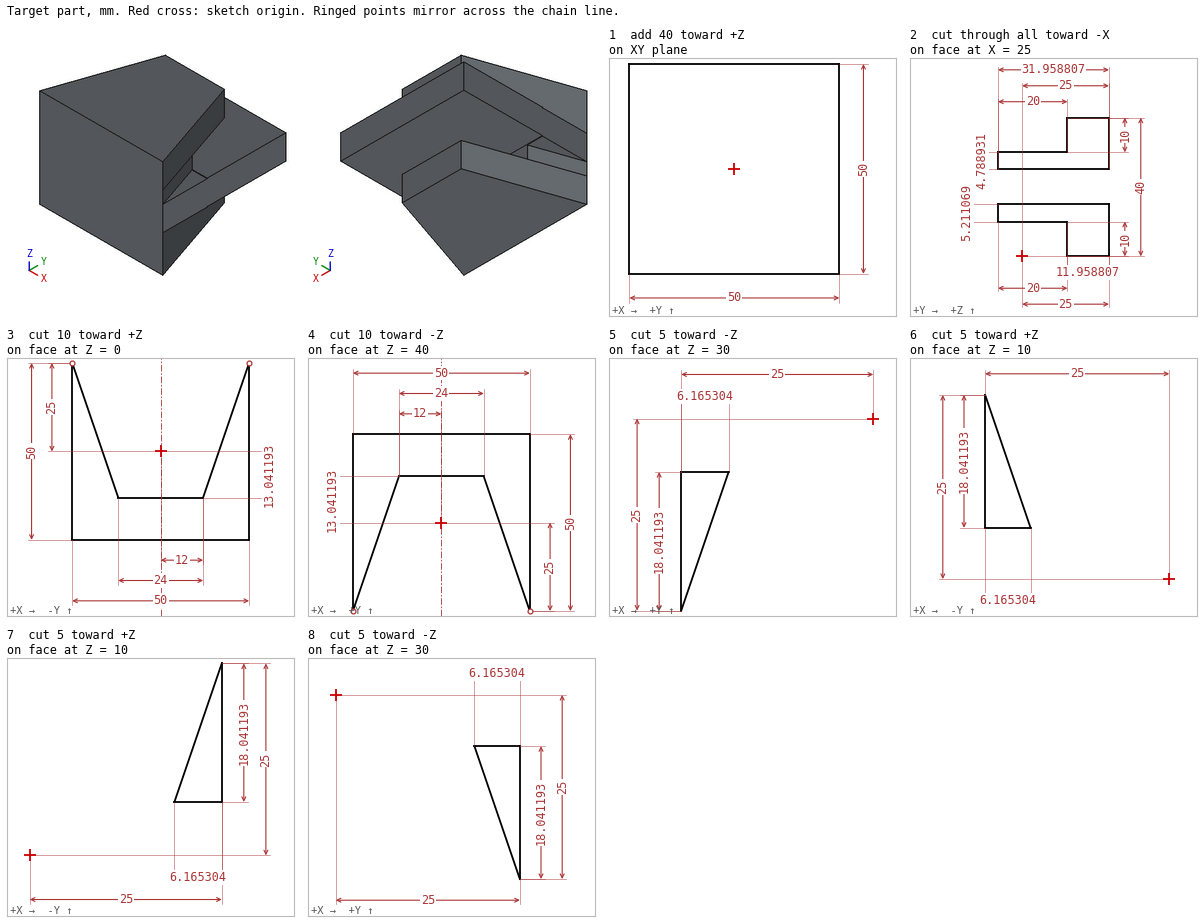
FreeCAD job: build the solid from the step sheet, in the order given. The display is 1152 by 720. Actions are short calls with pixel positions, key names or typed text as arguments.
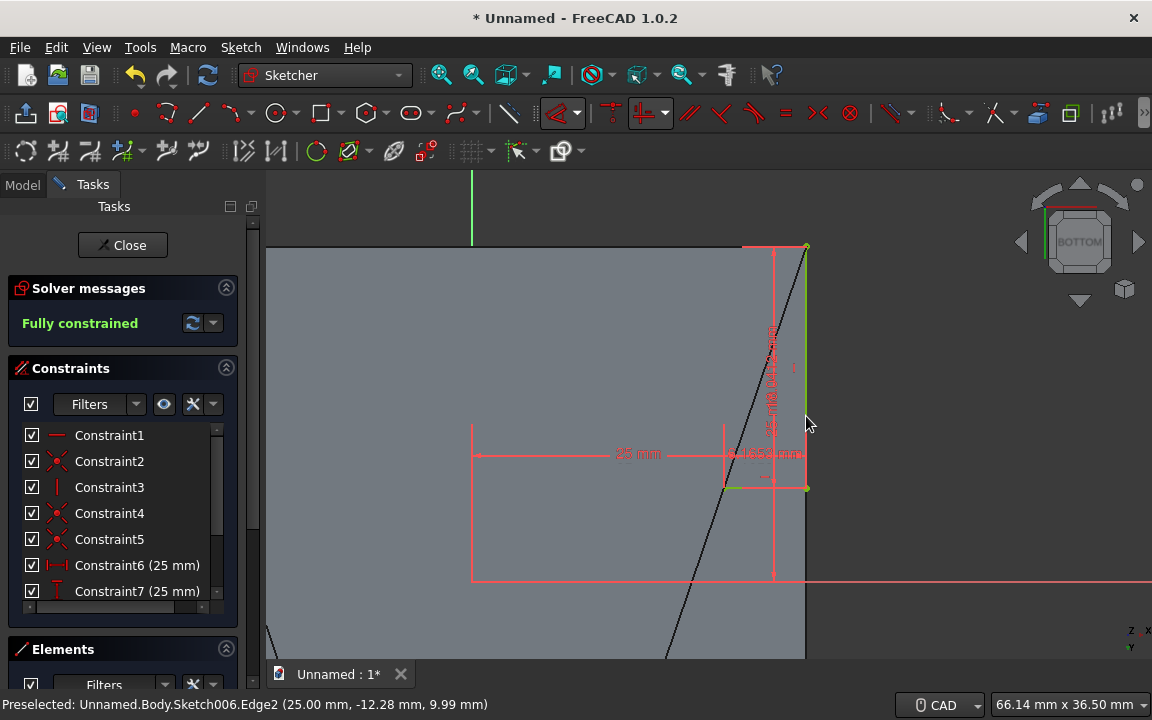
click(123, 245)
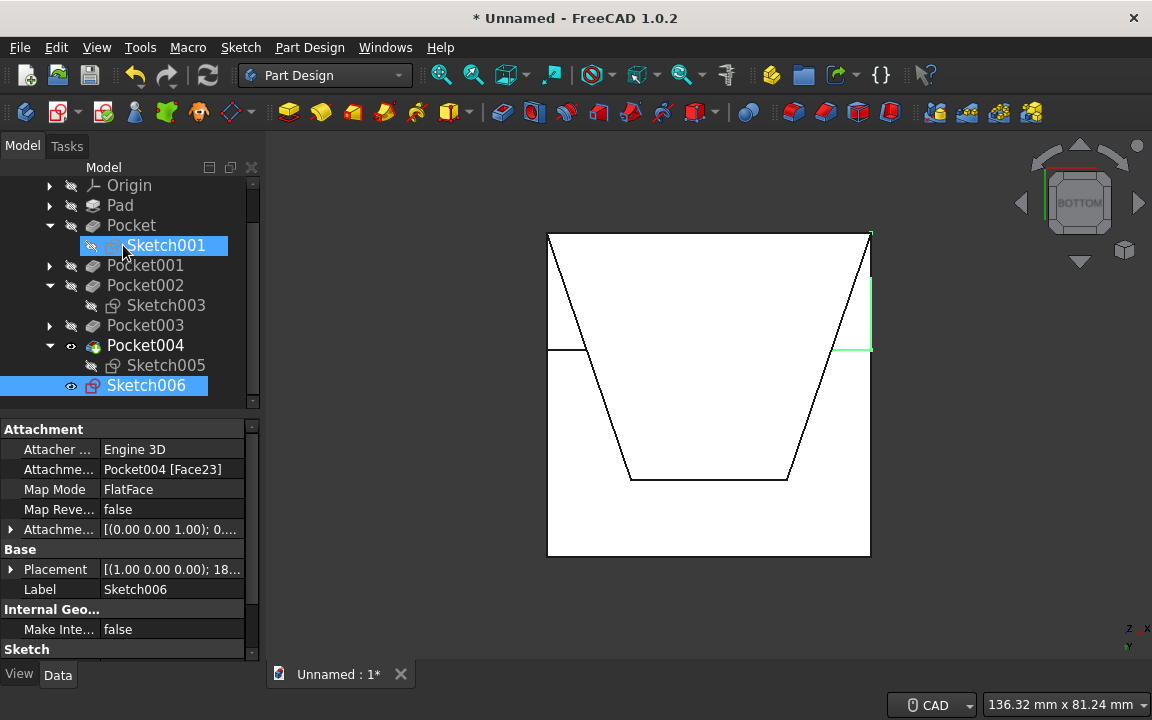
click(504, 112)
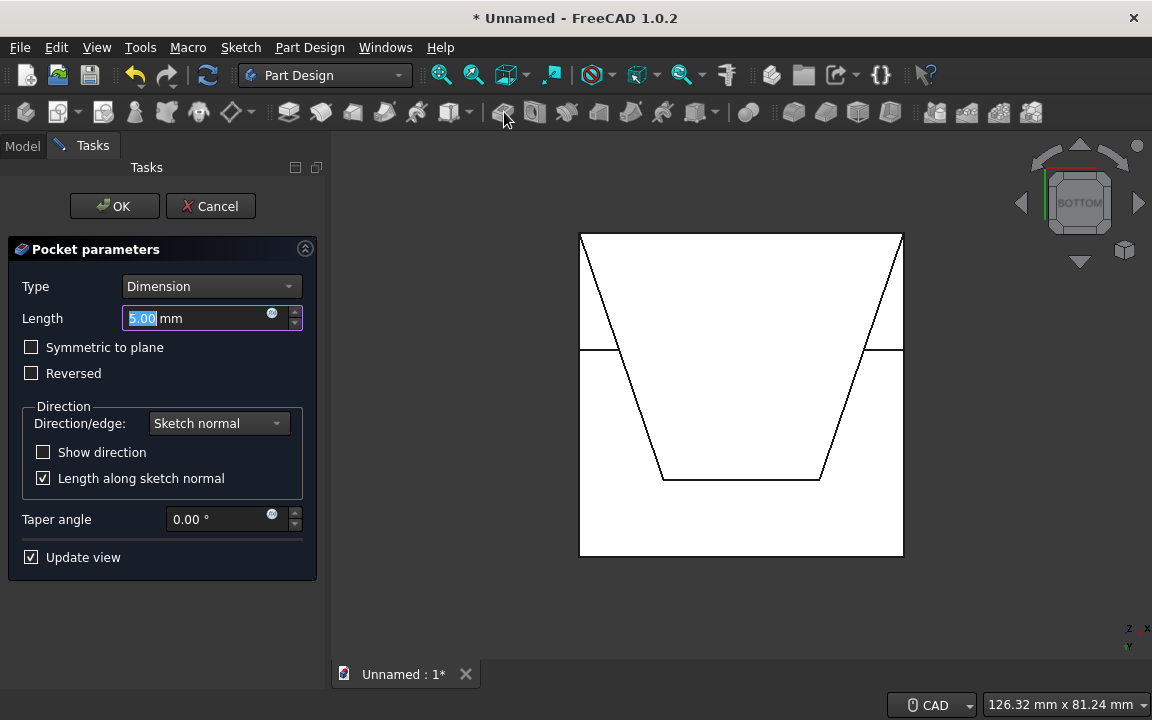
text(5)
key(Tab)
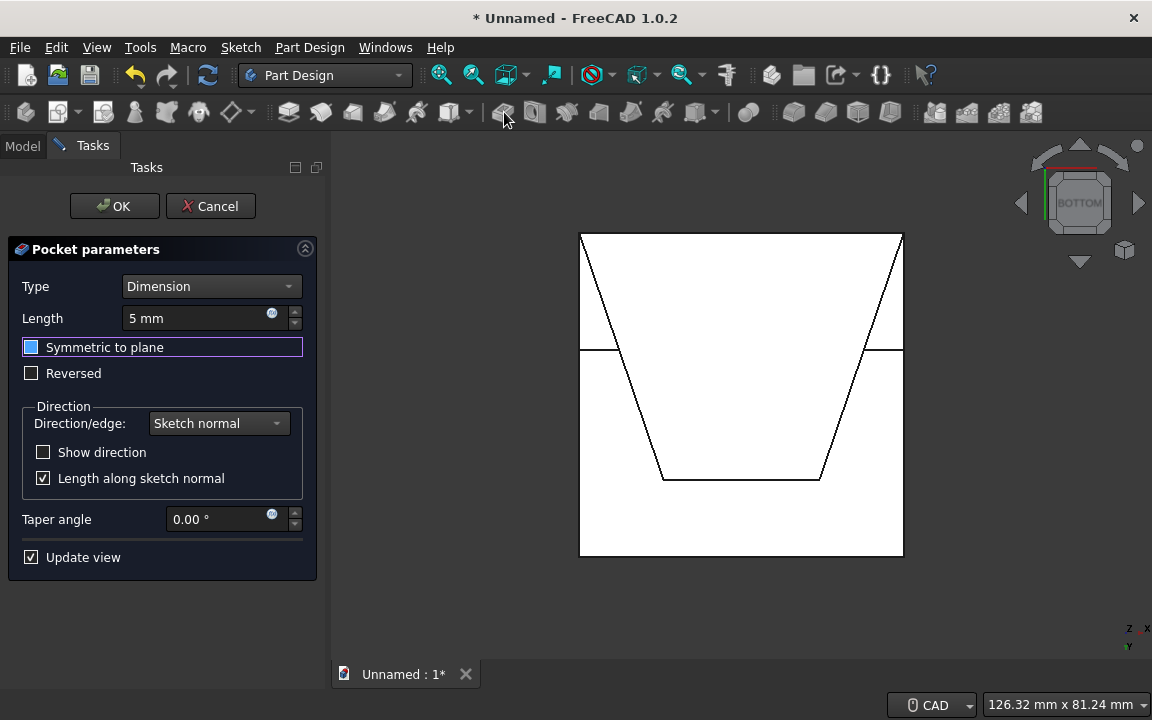
click(115, 206)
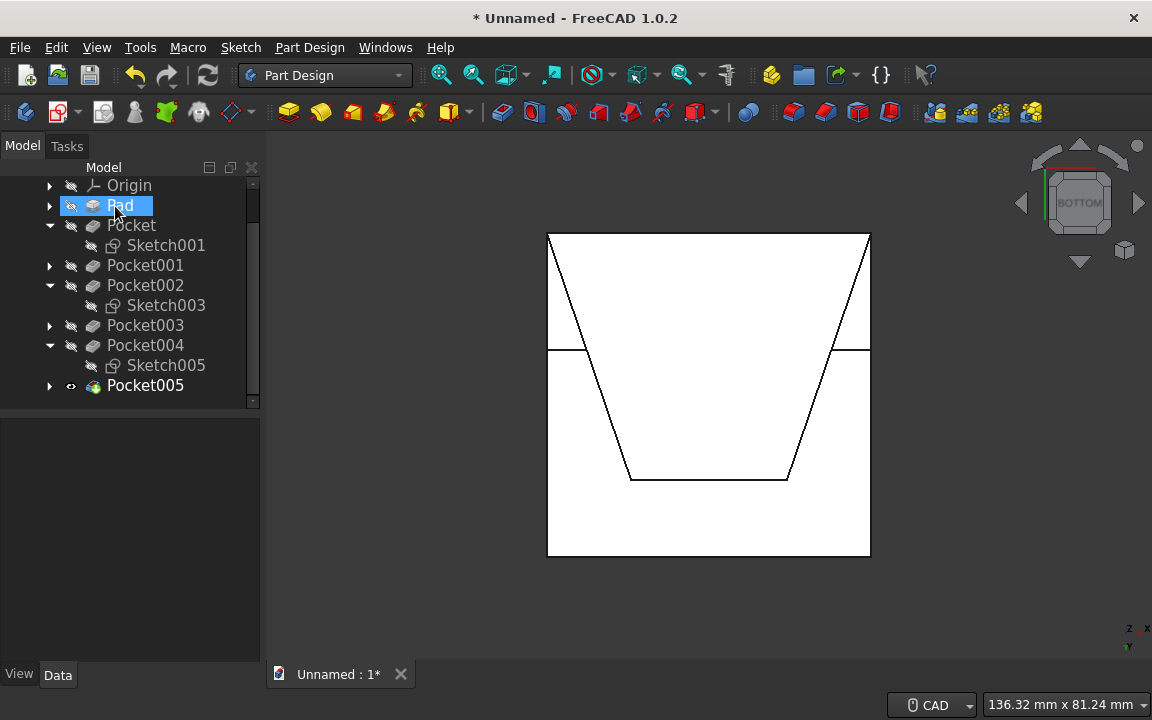
key(0)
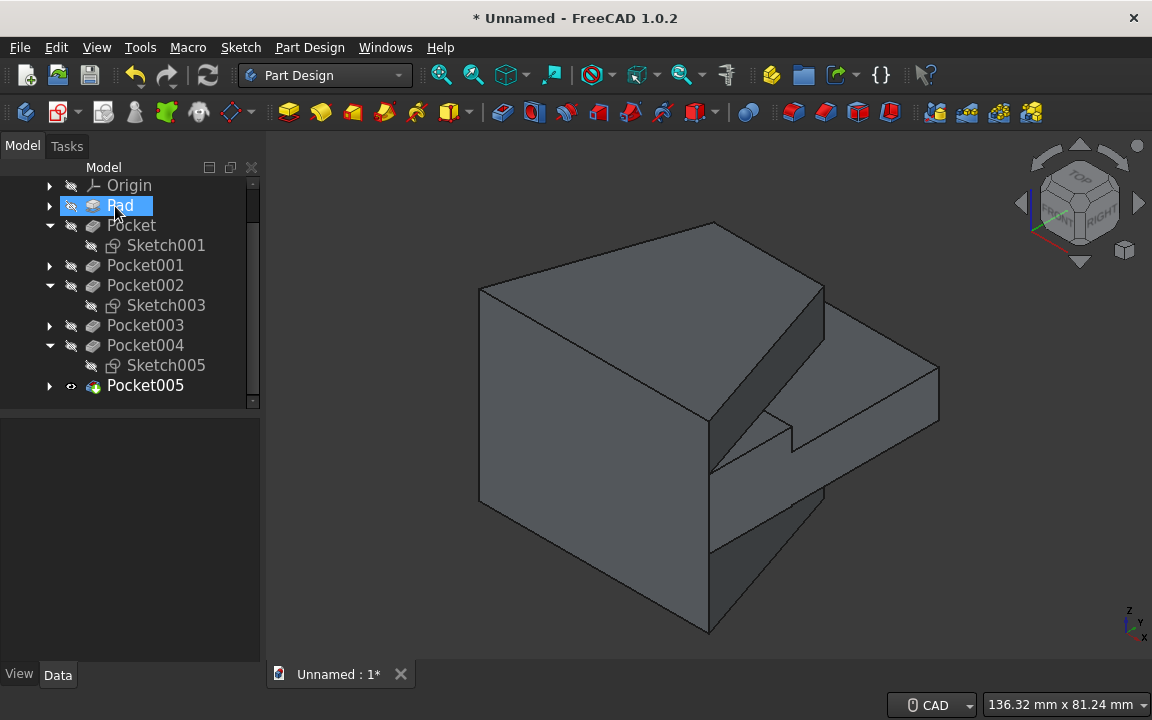
click(764, 430)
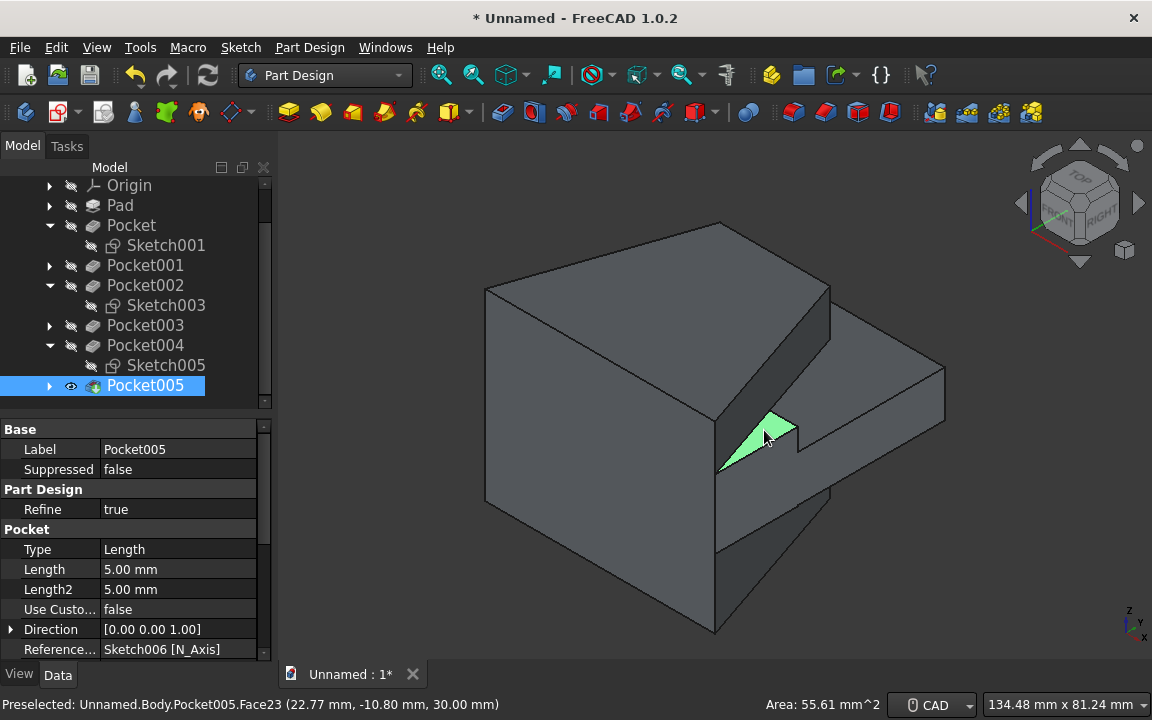
click(58, 112)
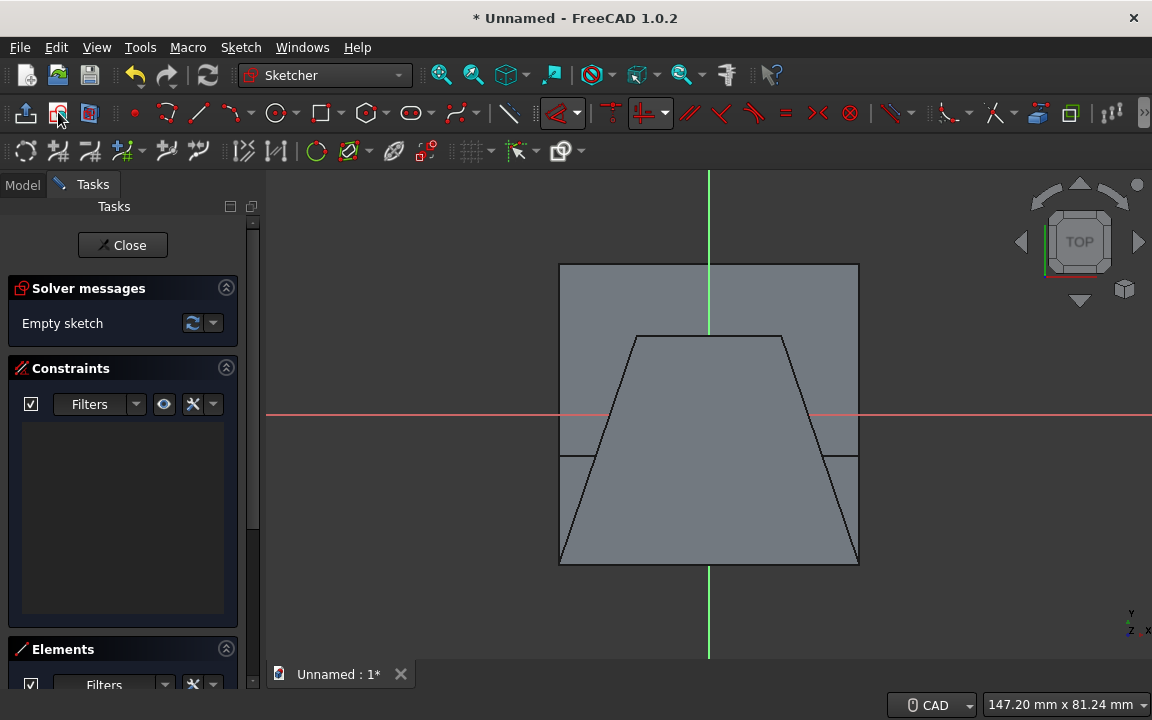
key(q)
key(s)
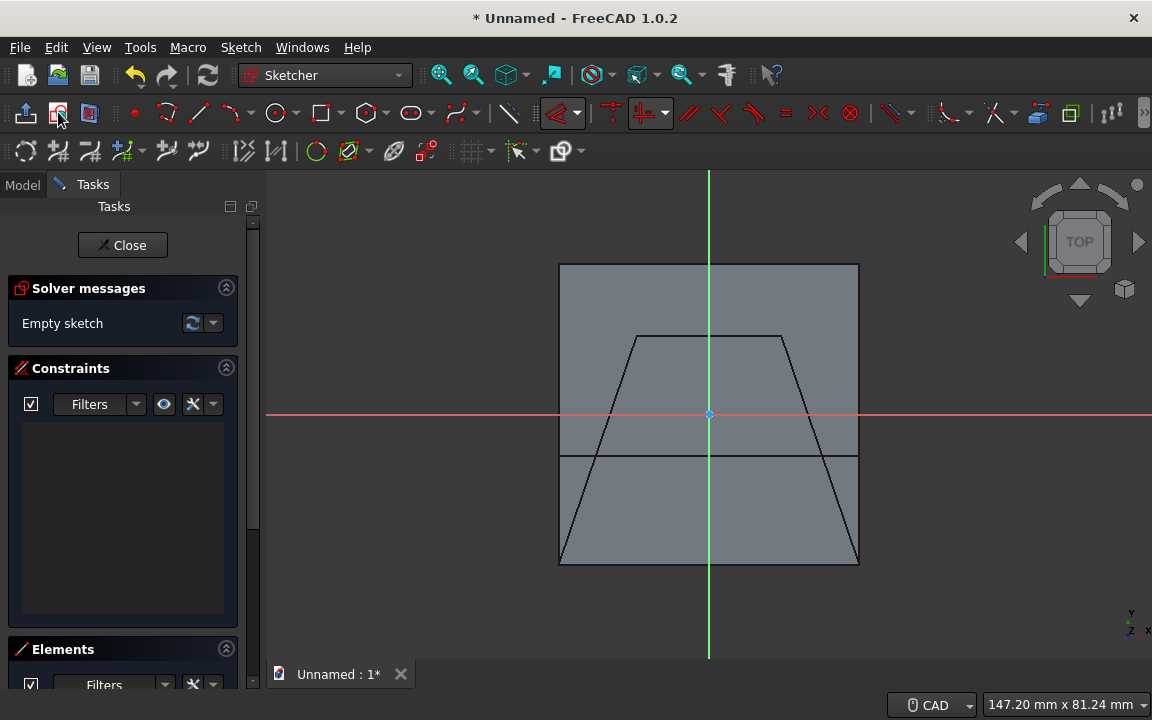
scroll(902, 551, up, 4)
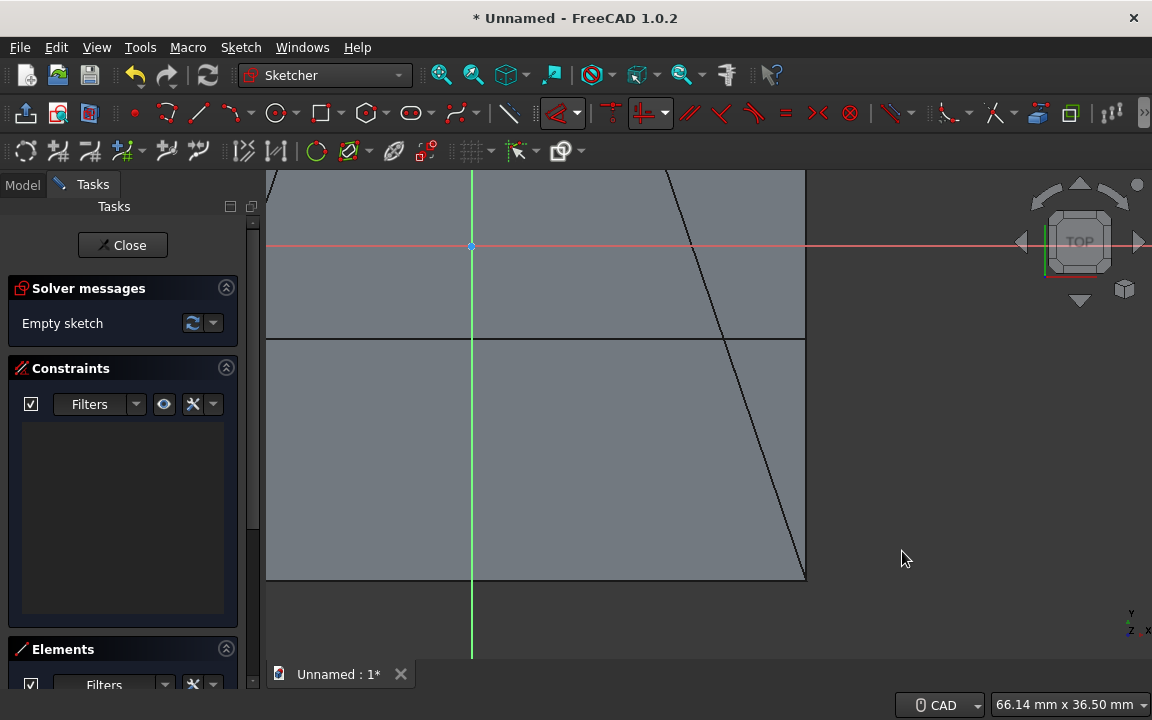
key(g)
key(m)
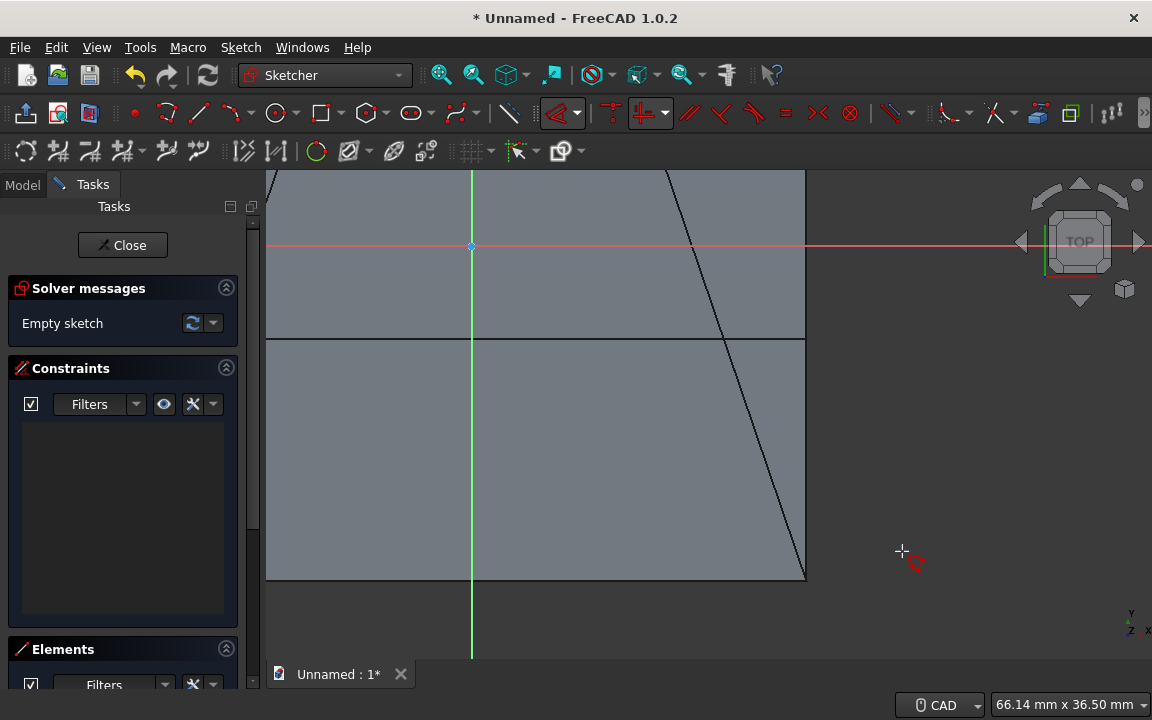
click(724, 339)
click(806, 581)
click(806, 339)
click(724, 340)
key(Escape)
key(Escape)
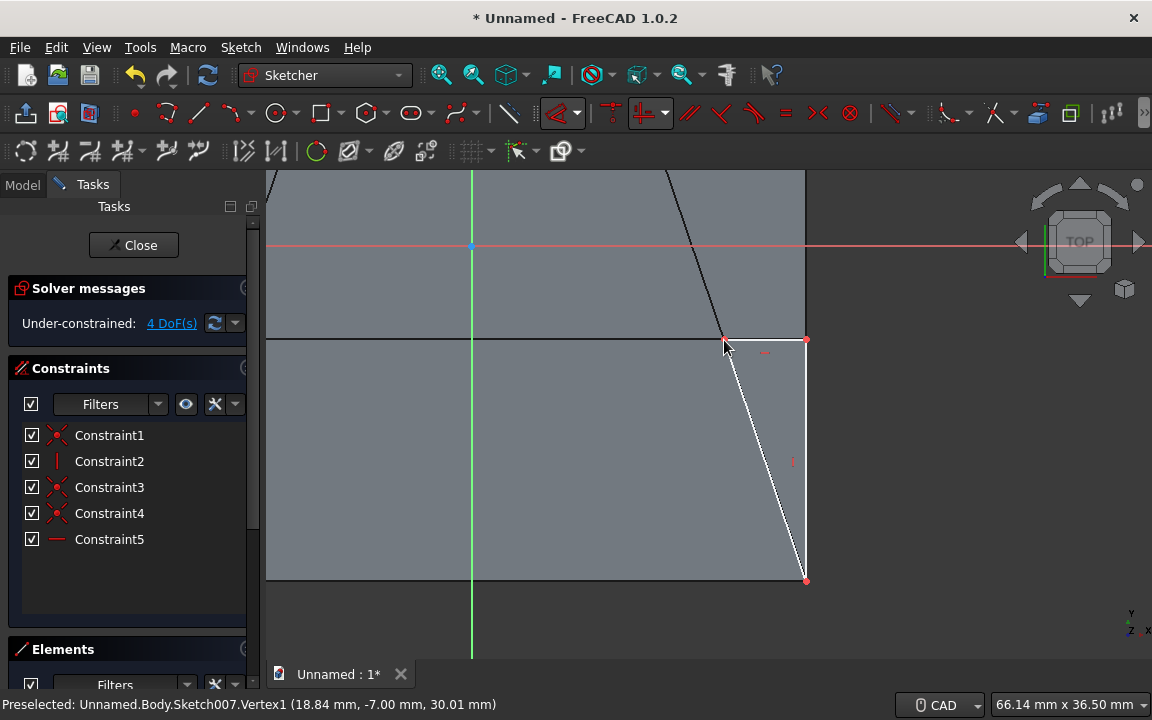
click(806, 582)